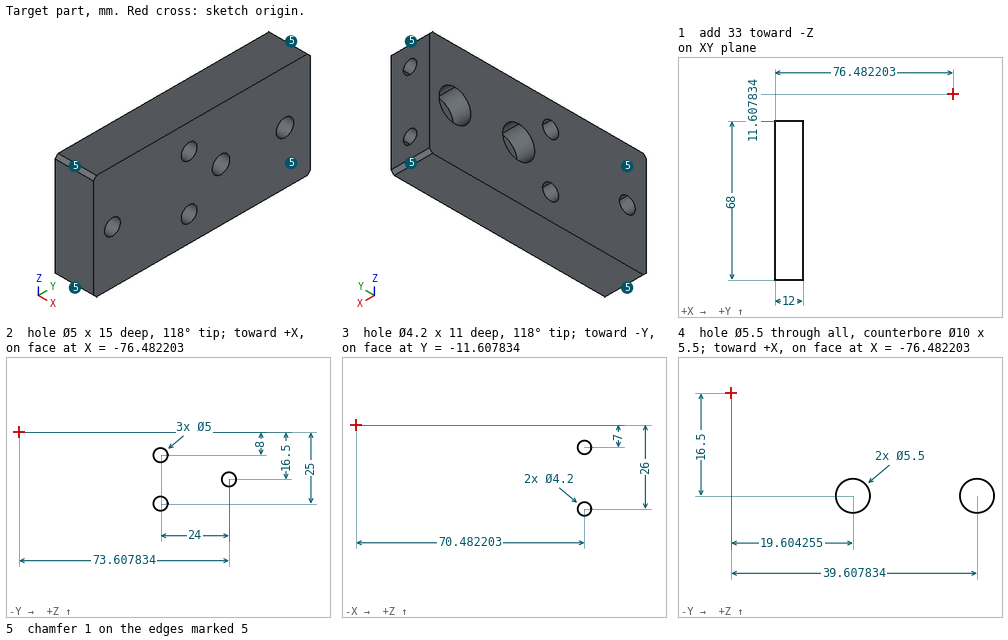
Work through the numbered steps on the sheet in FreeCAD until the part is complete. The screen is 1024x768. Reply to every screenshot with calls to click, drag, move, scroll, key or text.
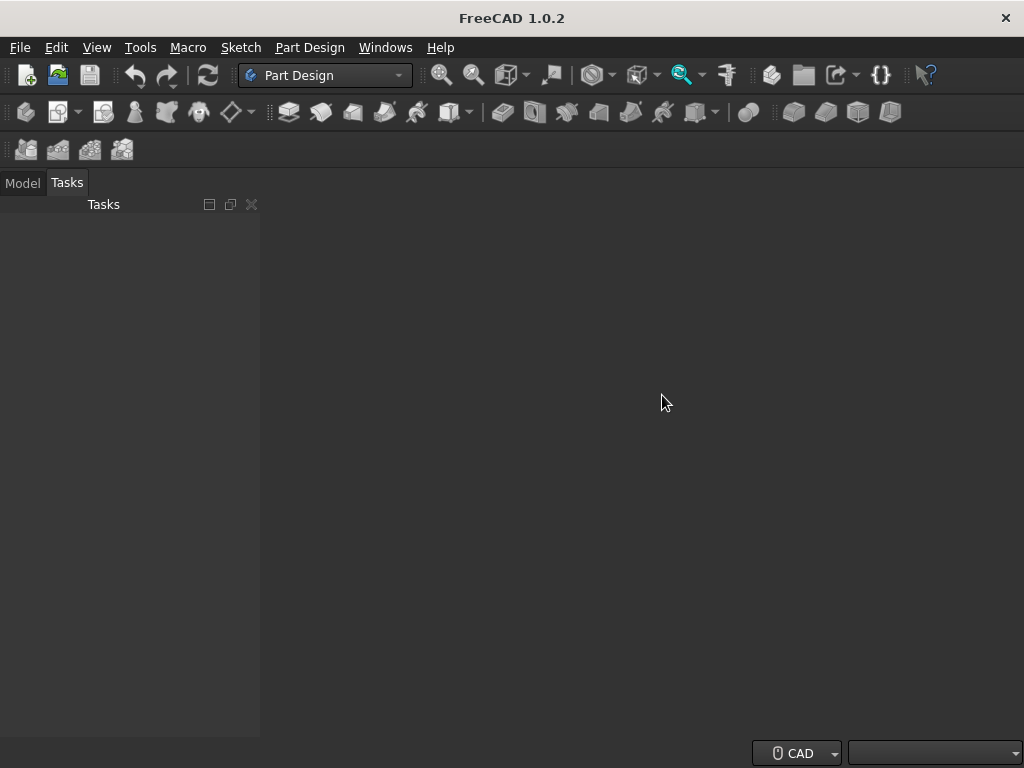
key(ctrl+n)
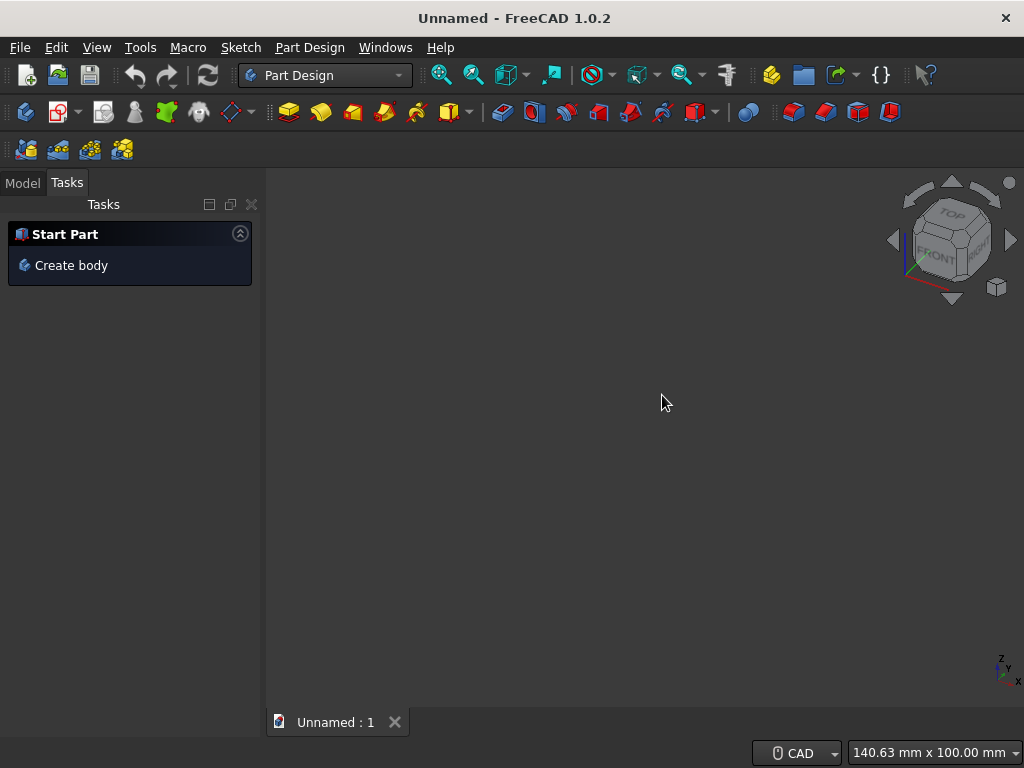
click(58, 112)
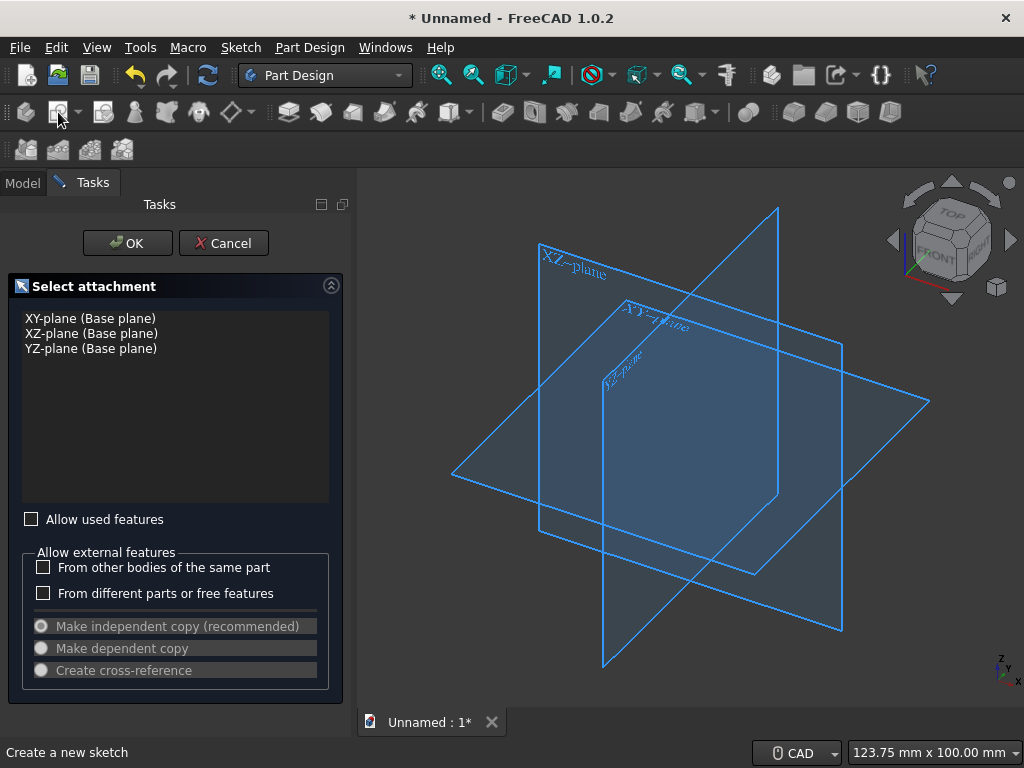
click(82, 318)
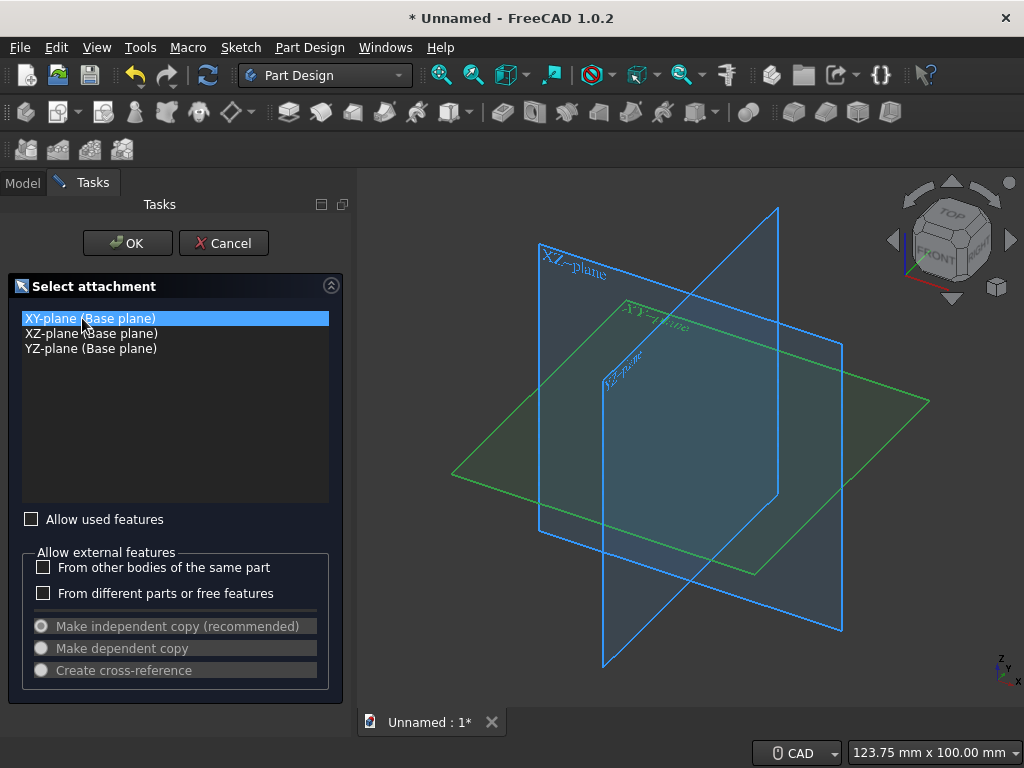
click(128, 243)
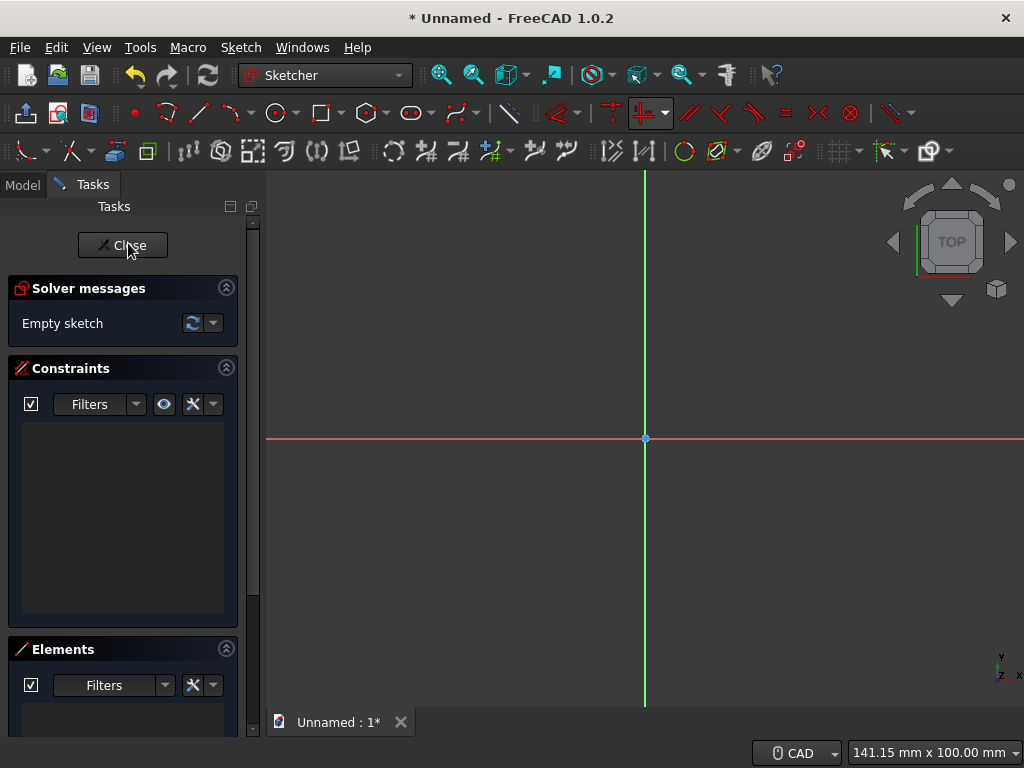
scroll(855, 198, down, 2)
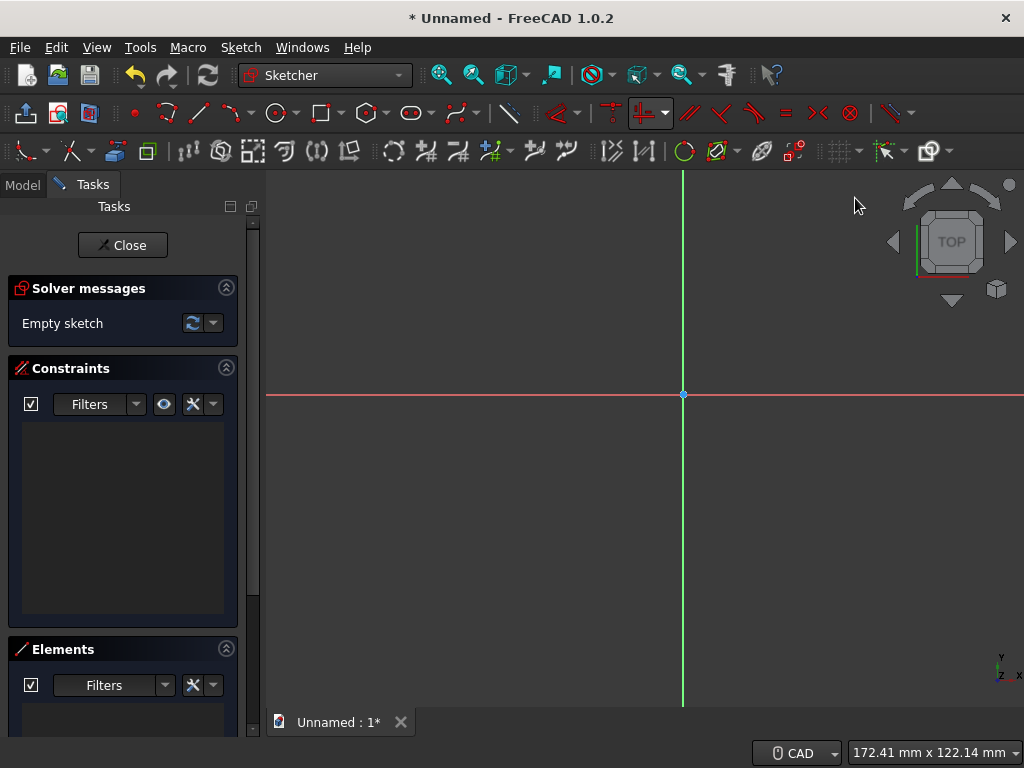
key(g)
key(r)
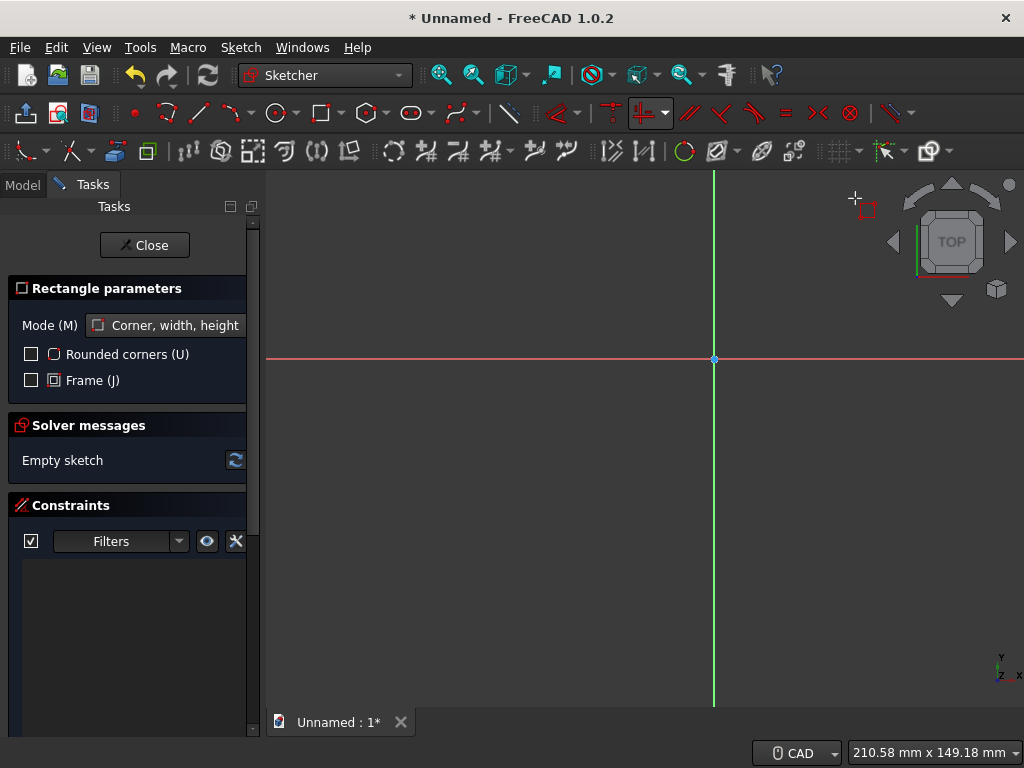
click(439, 401)
click(482, 646)
key(Escape)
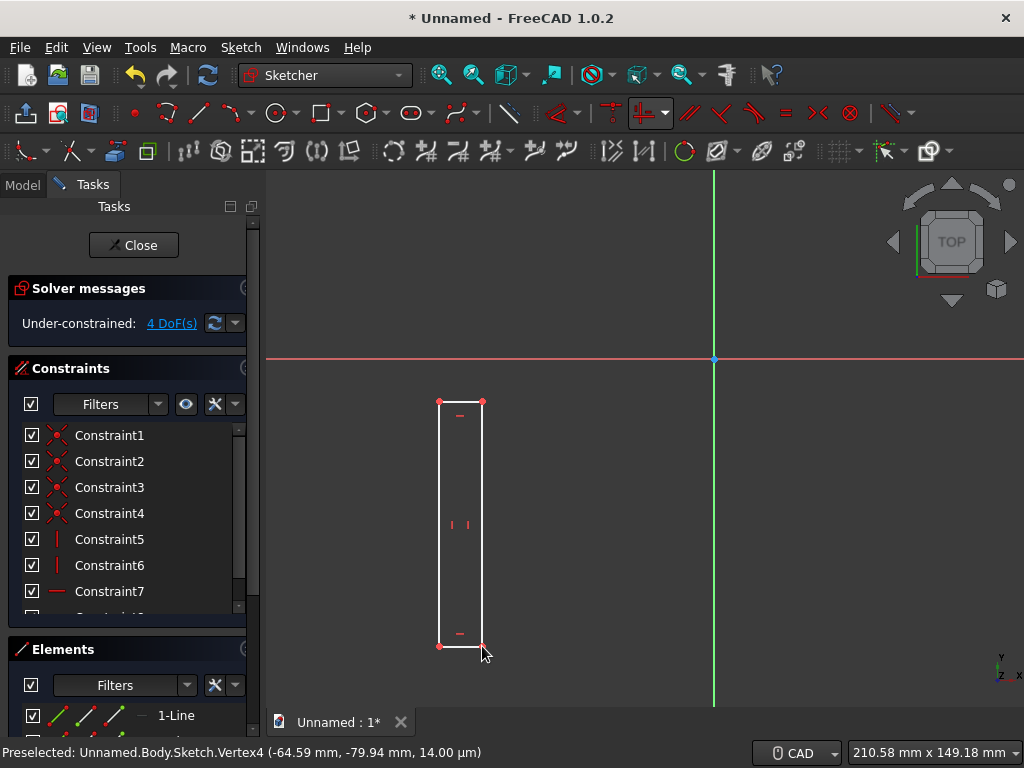
key(d)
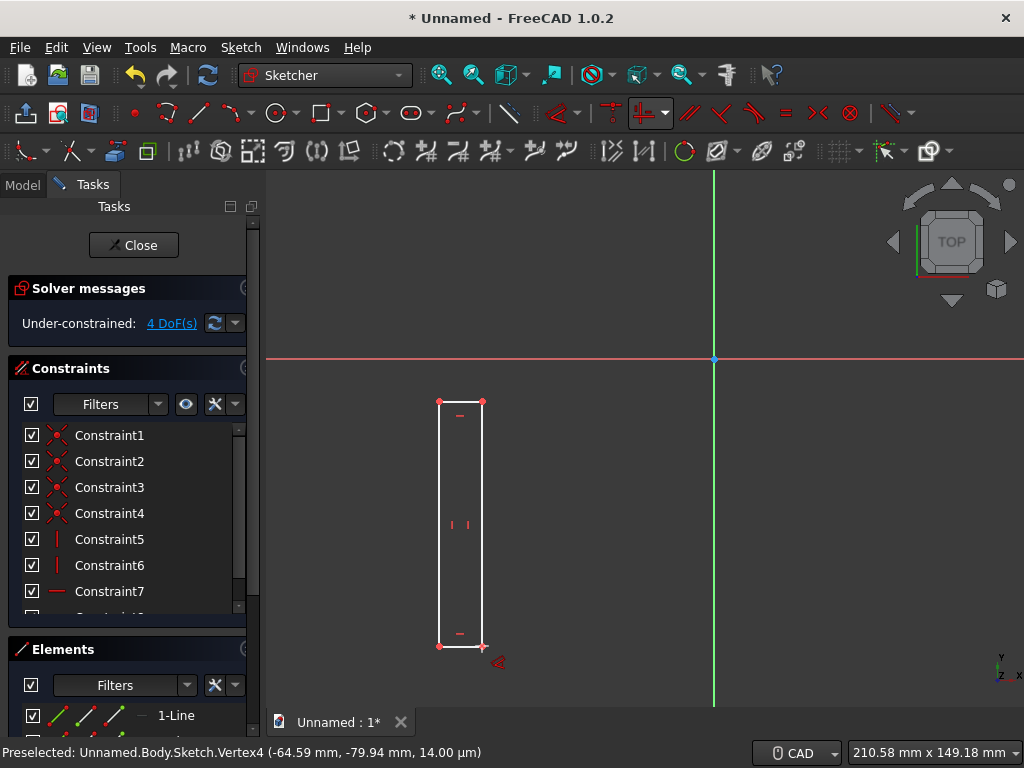
click(439, 475)
click(405, 524)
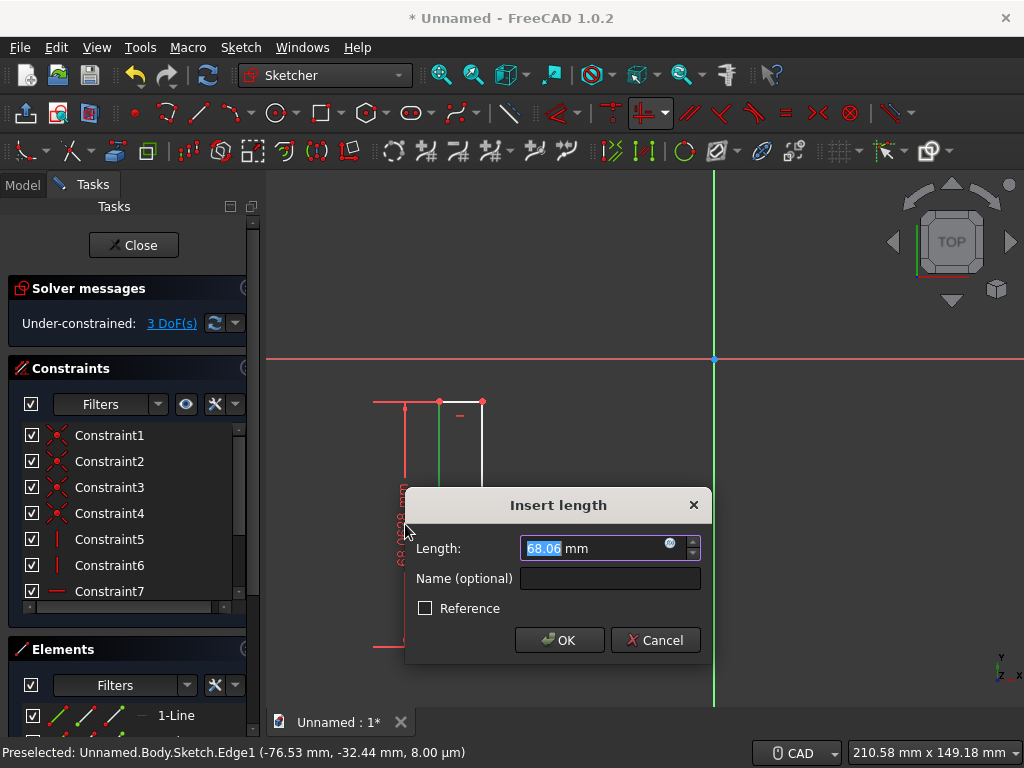
text(68)
key(Return)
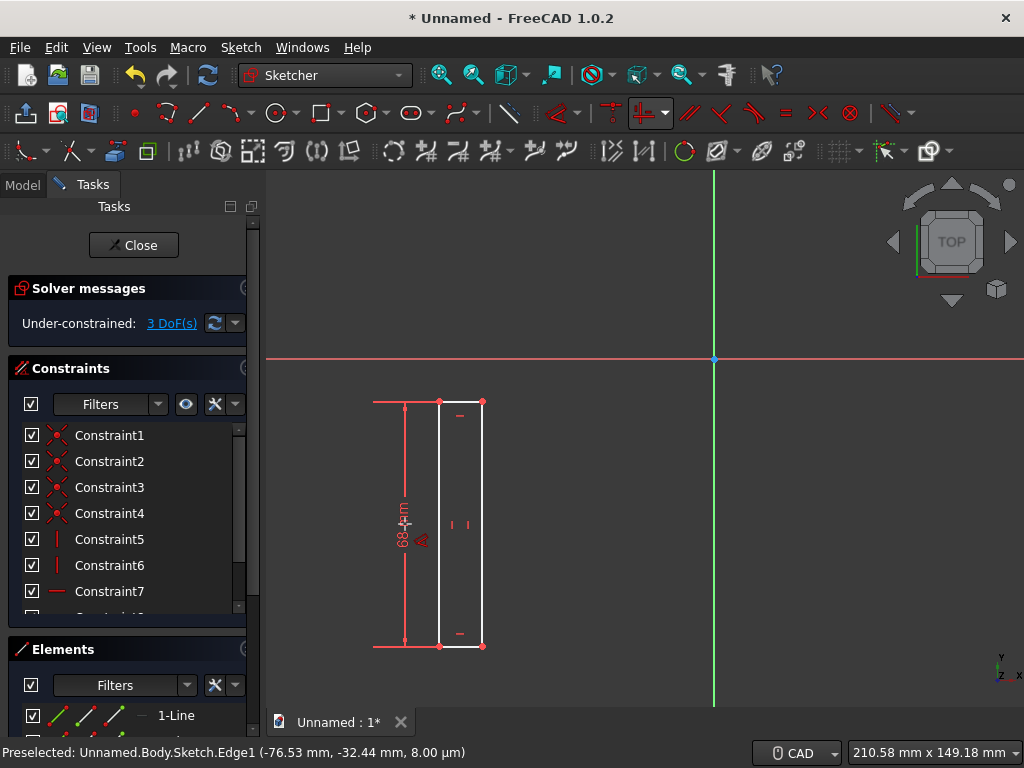
click(452, 647)
click(461, 613)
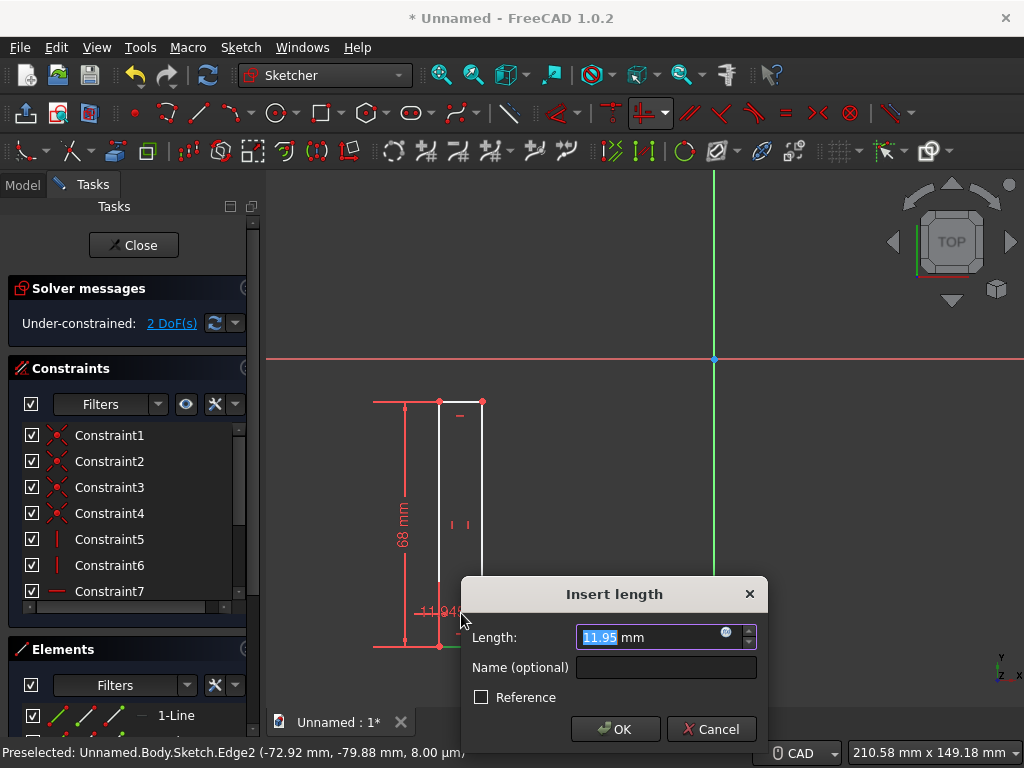
text(12)
key(Return)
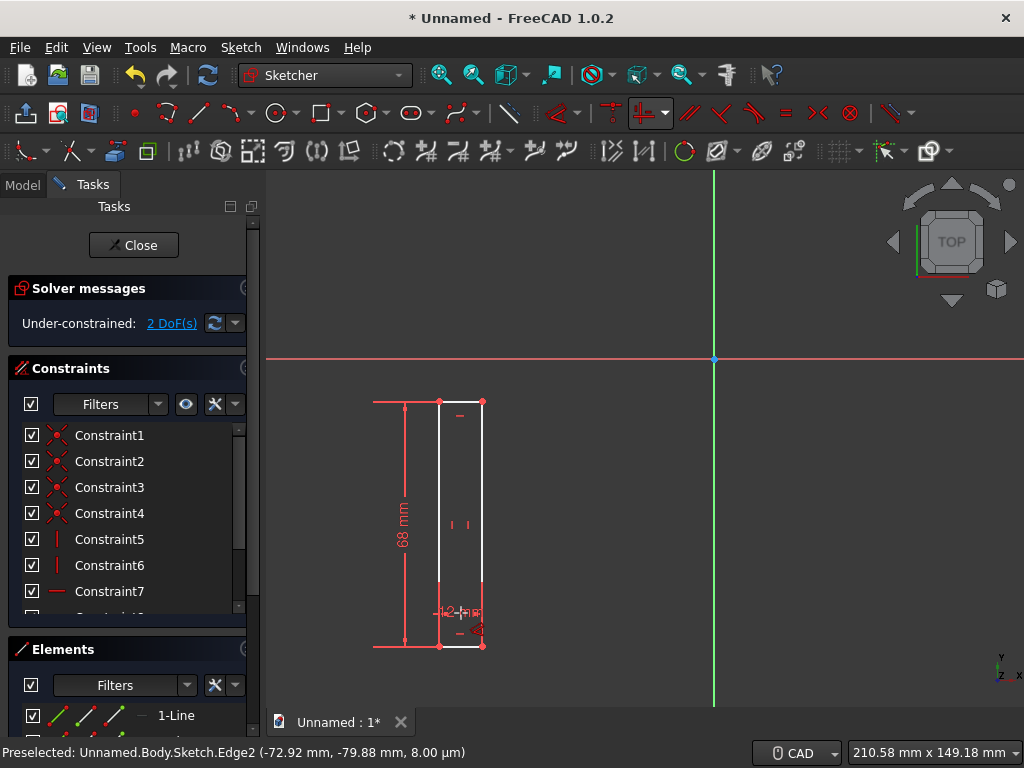
click(439, 402)
click(577, 325)